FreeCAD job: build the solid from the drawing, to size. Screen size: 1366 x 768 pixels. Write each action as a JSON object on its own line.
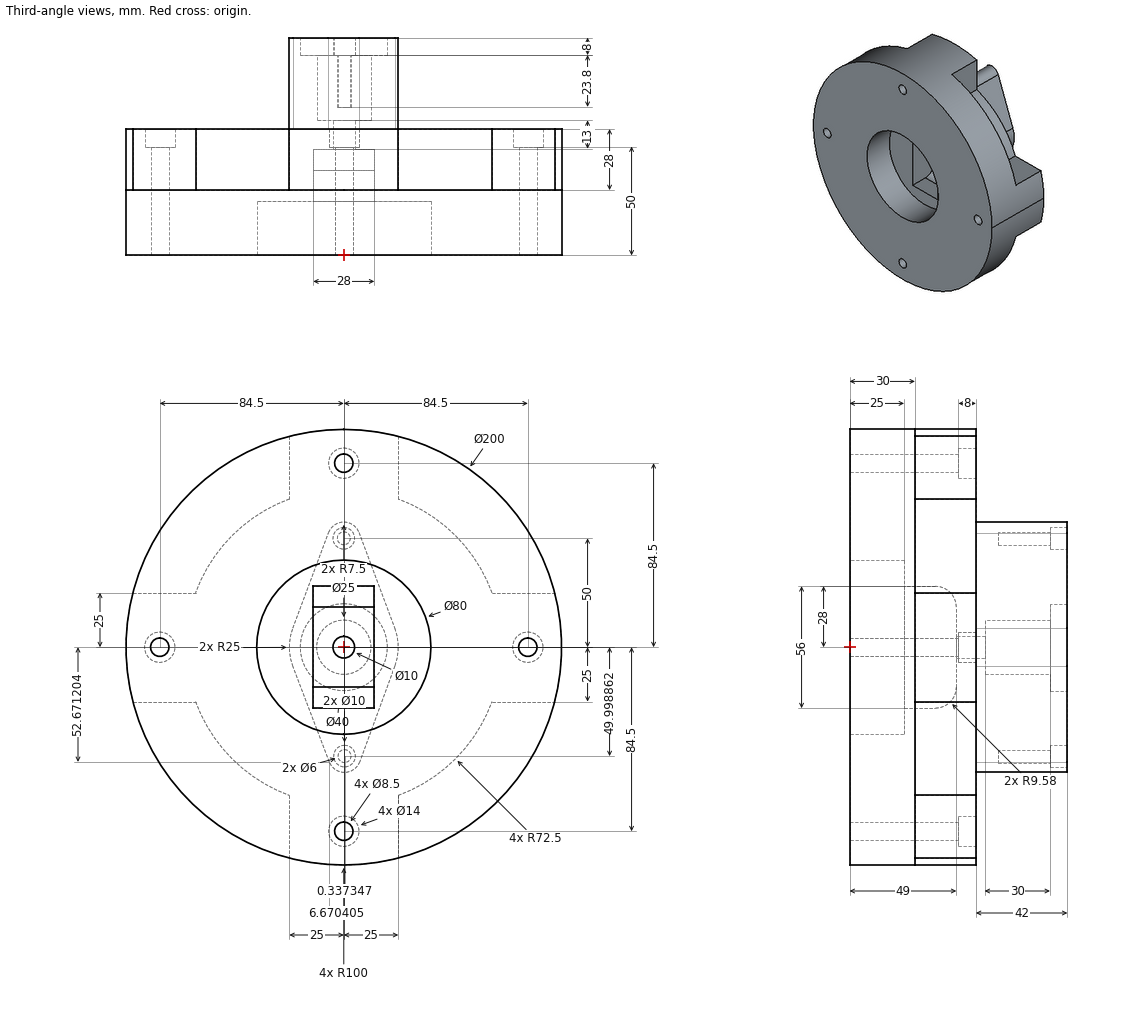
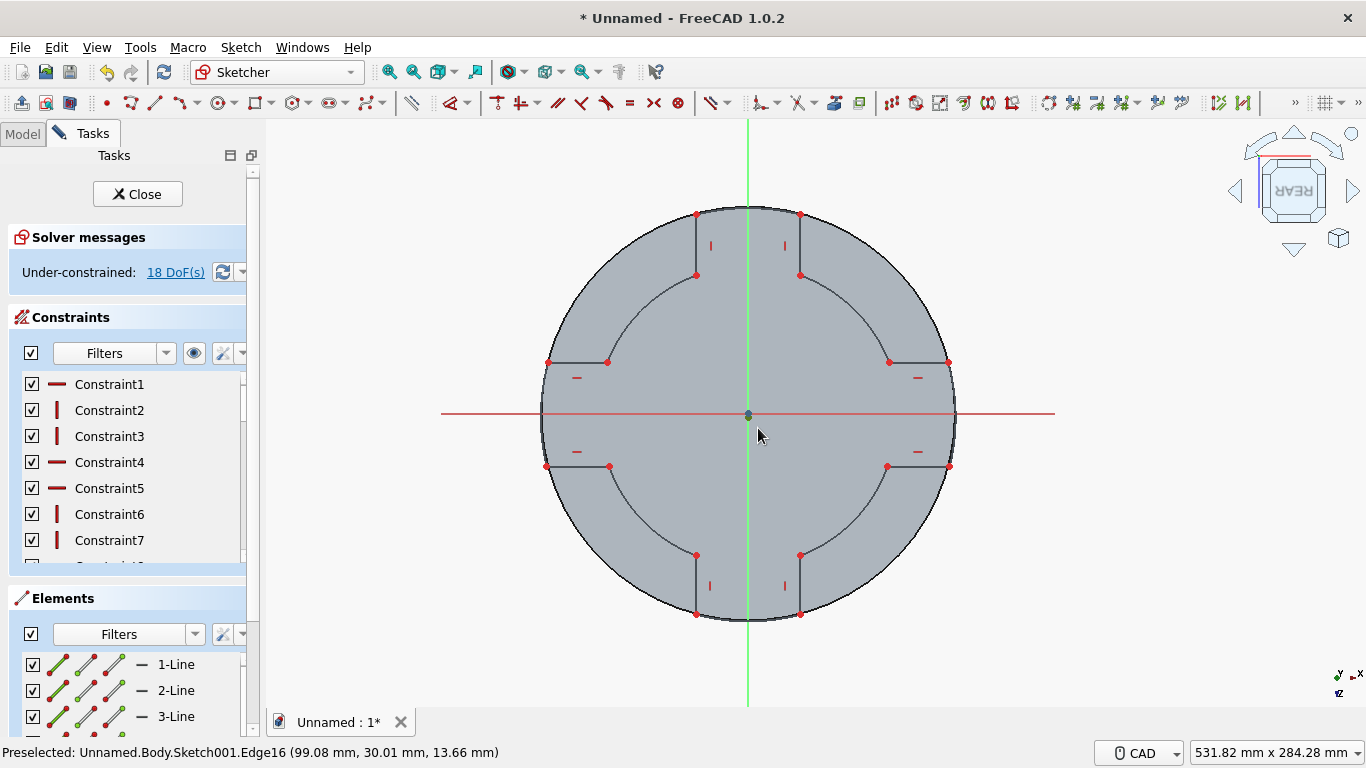
{"action": "left_click", "coordinate": [498, 104]}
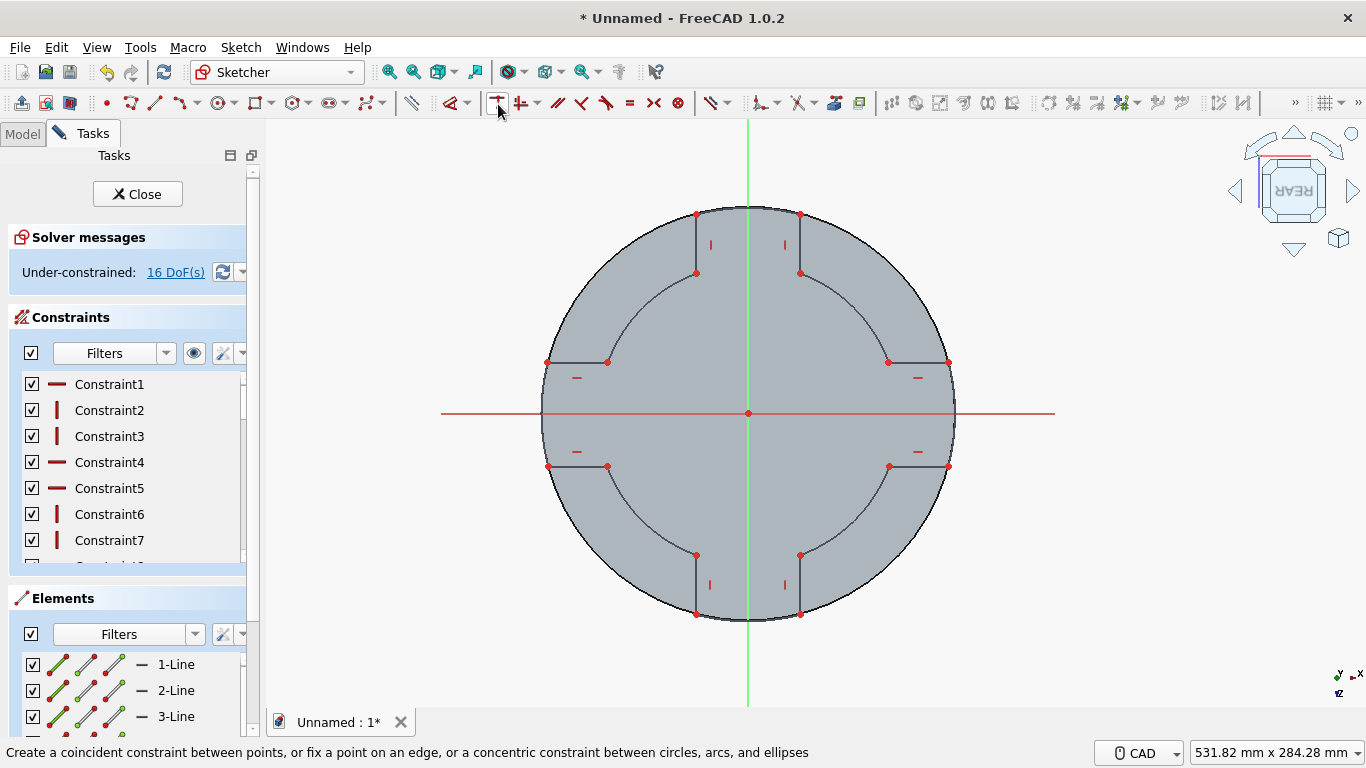
{"action": "left_click", "coordinate": [871, 328]}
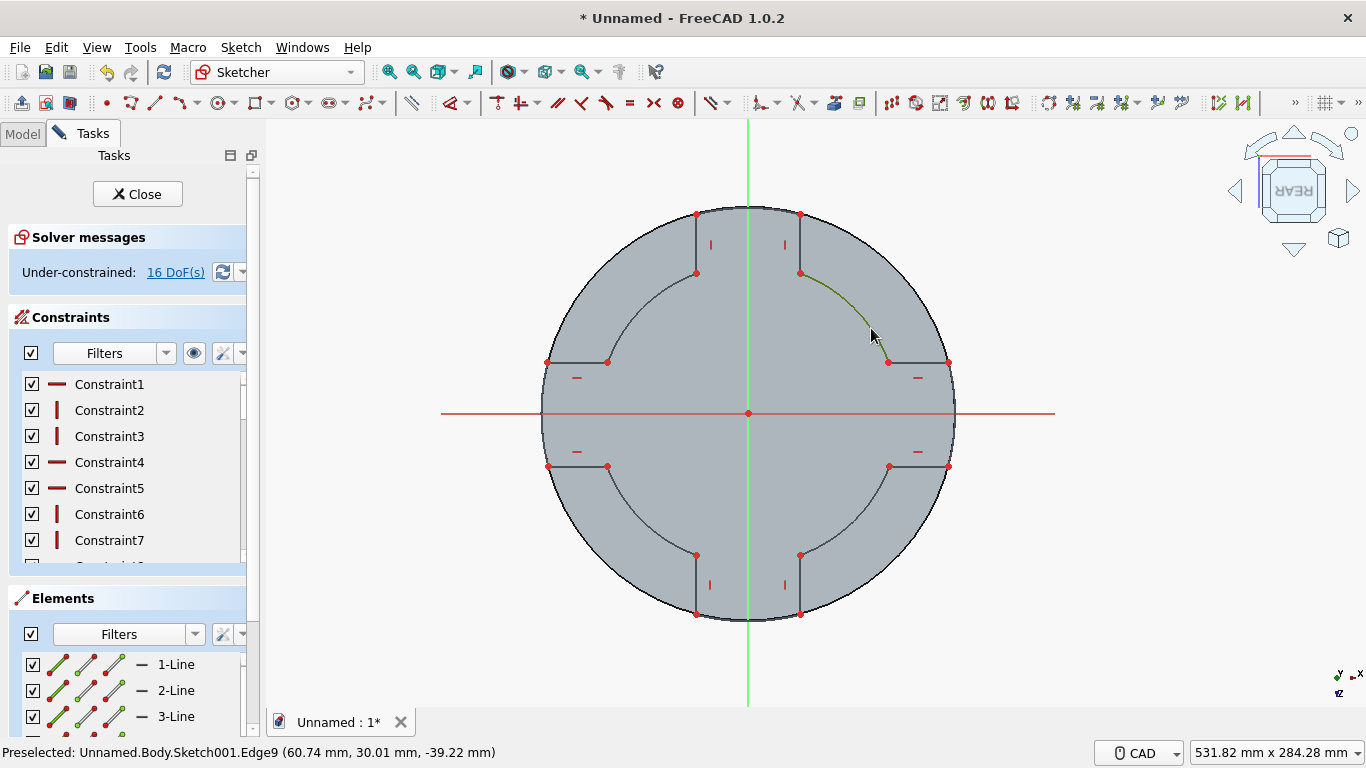
{"action": "left_click", "coordinate": [662, 292]}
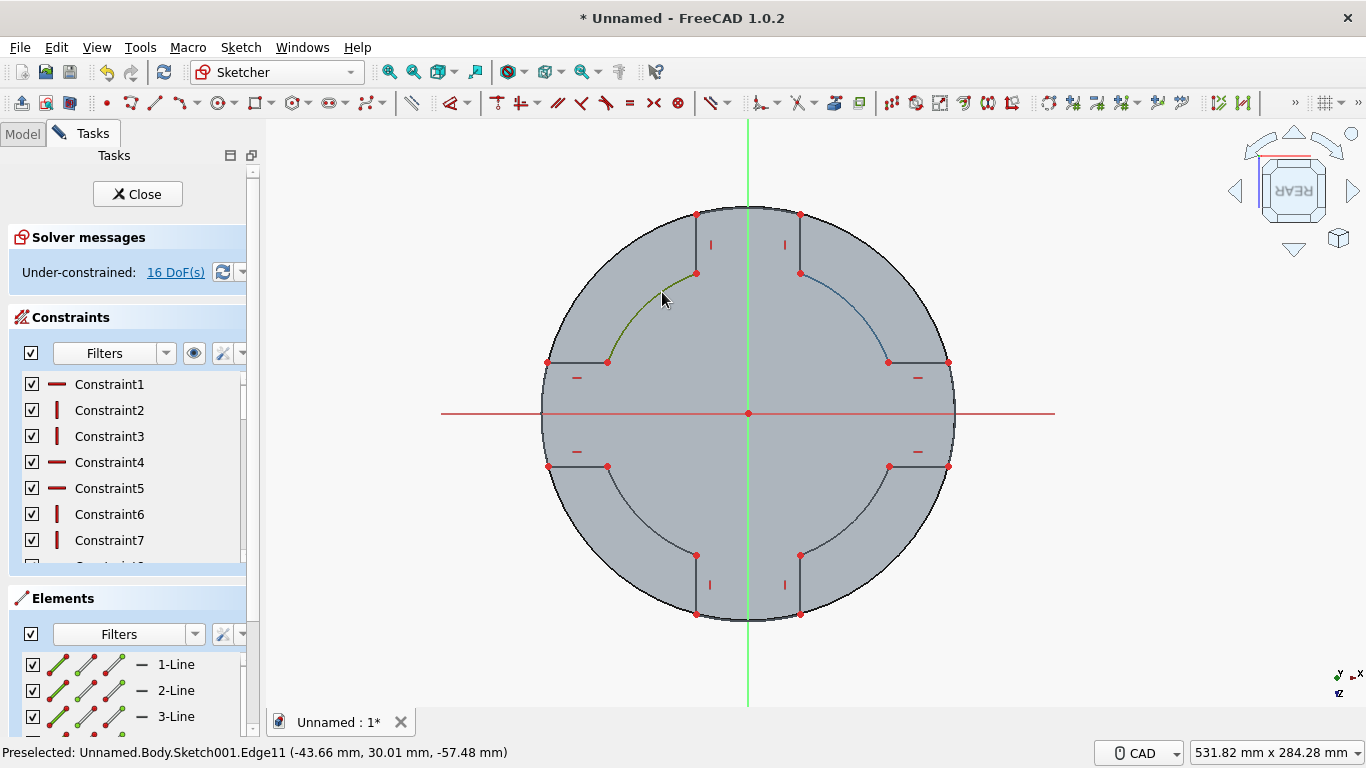
{"action": "left_click", "coordinate": [625, 501]}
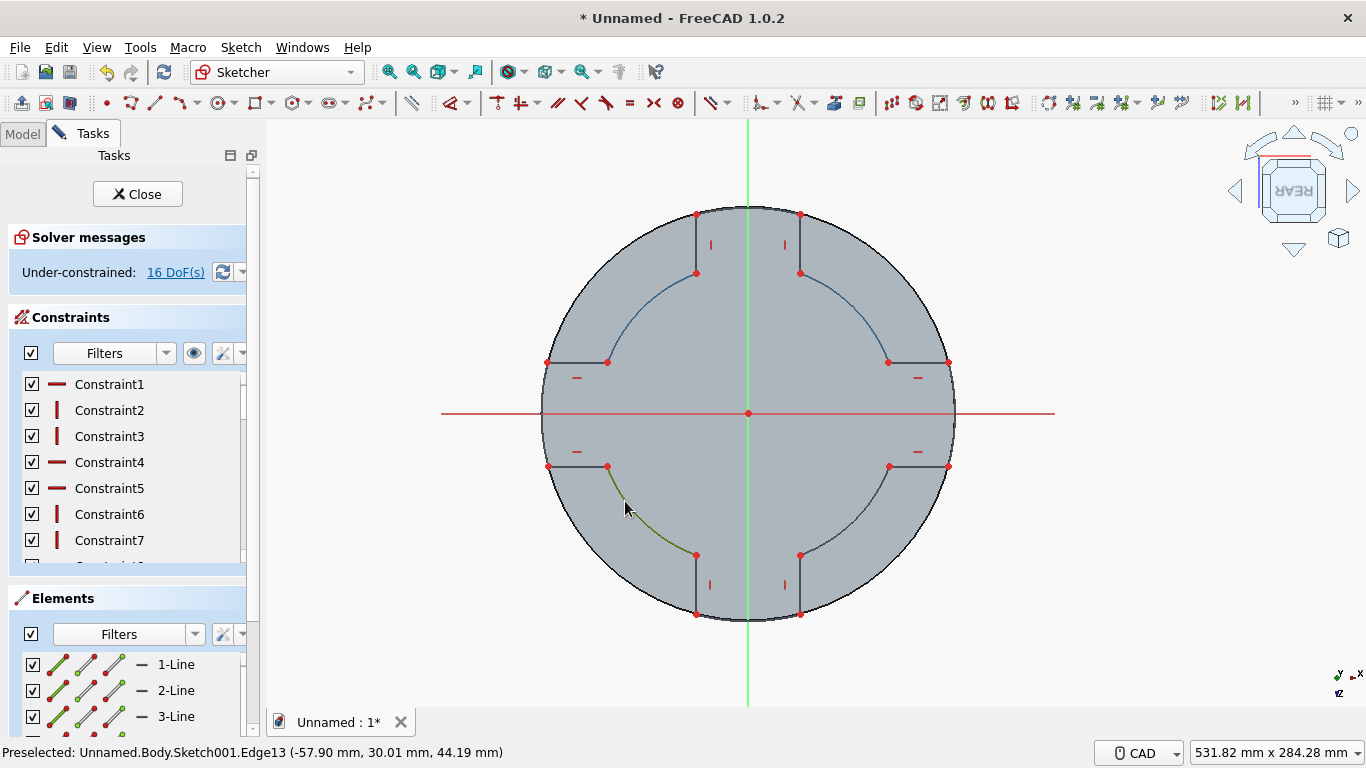
{"action": "left_click", "coordinate": [835, 537]}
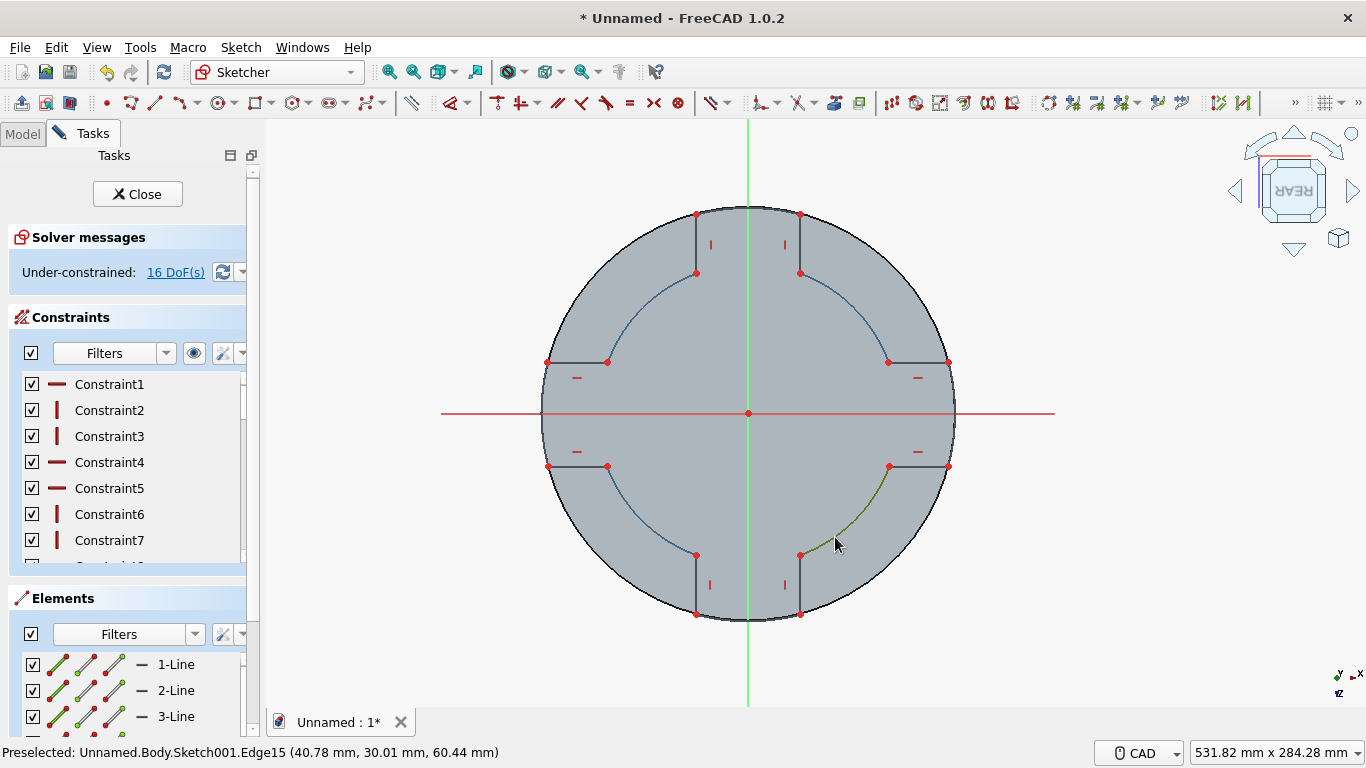
{"action": "key", "text": "e"}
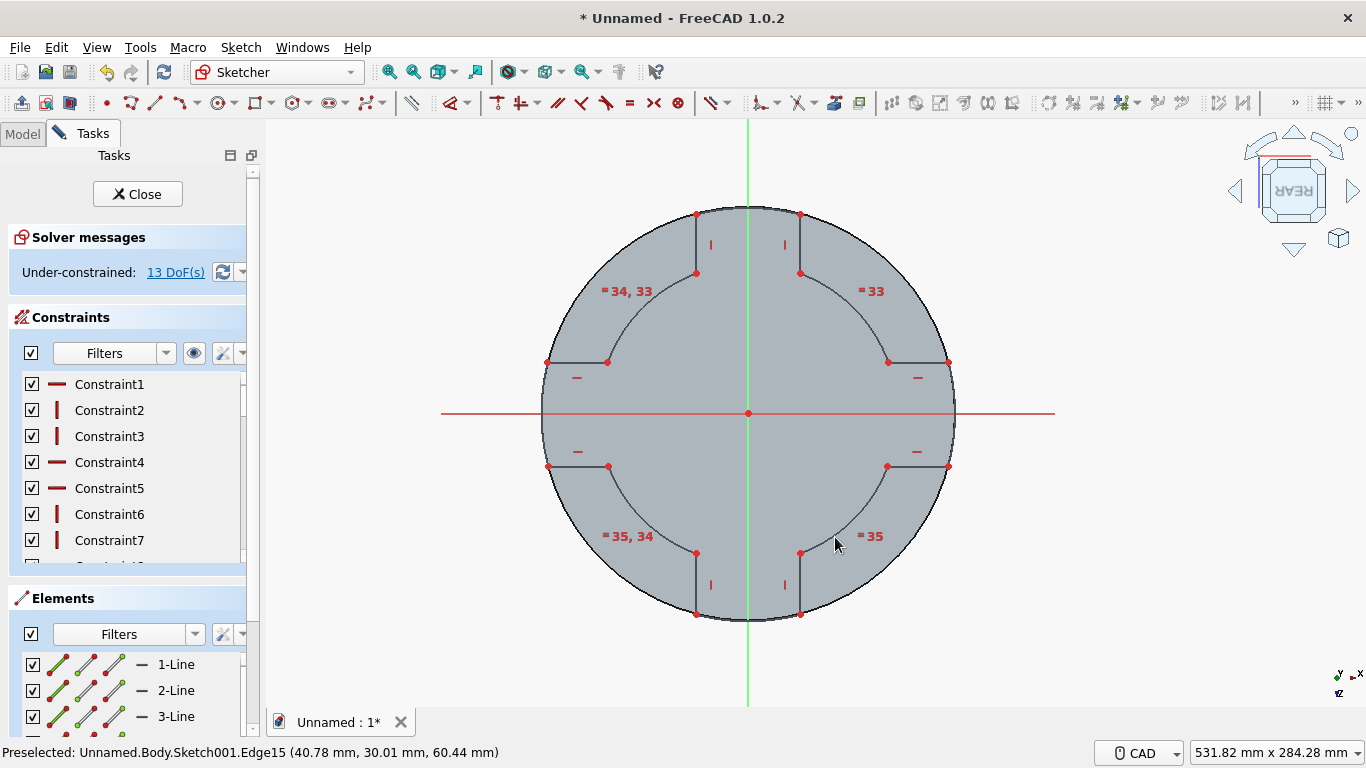
{"action": "left_click", "coordinate": [769, 209]}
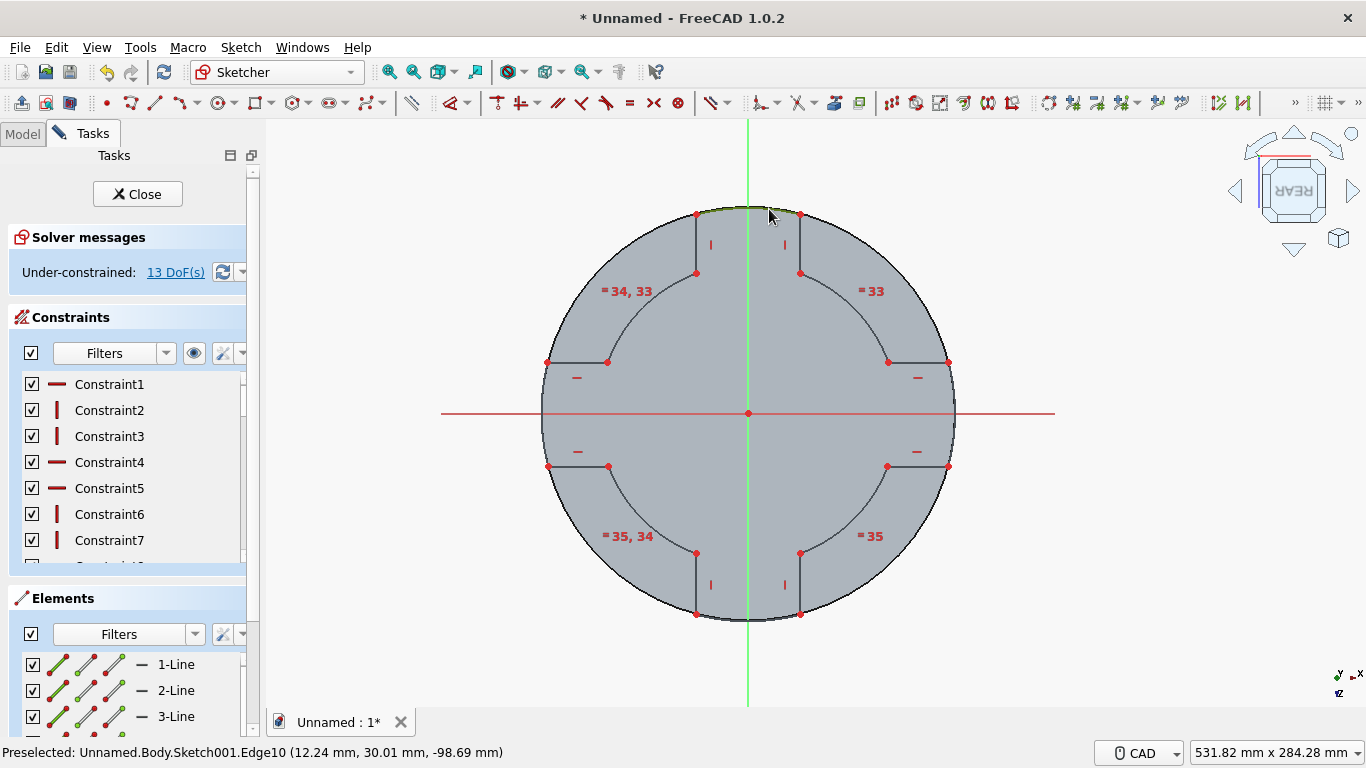
{"action": "left_click", "coordinate": [542, 394]}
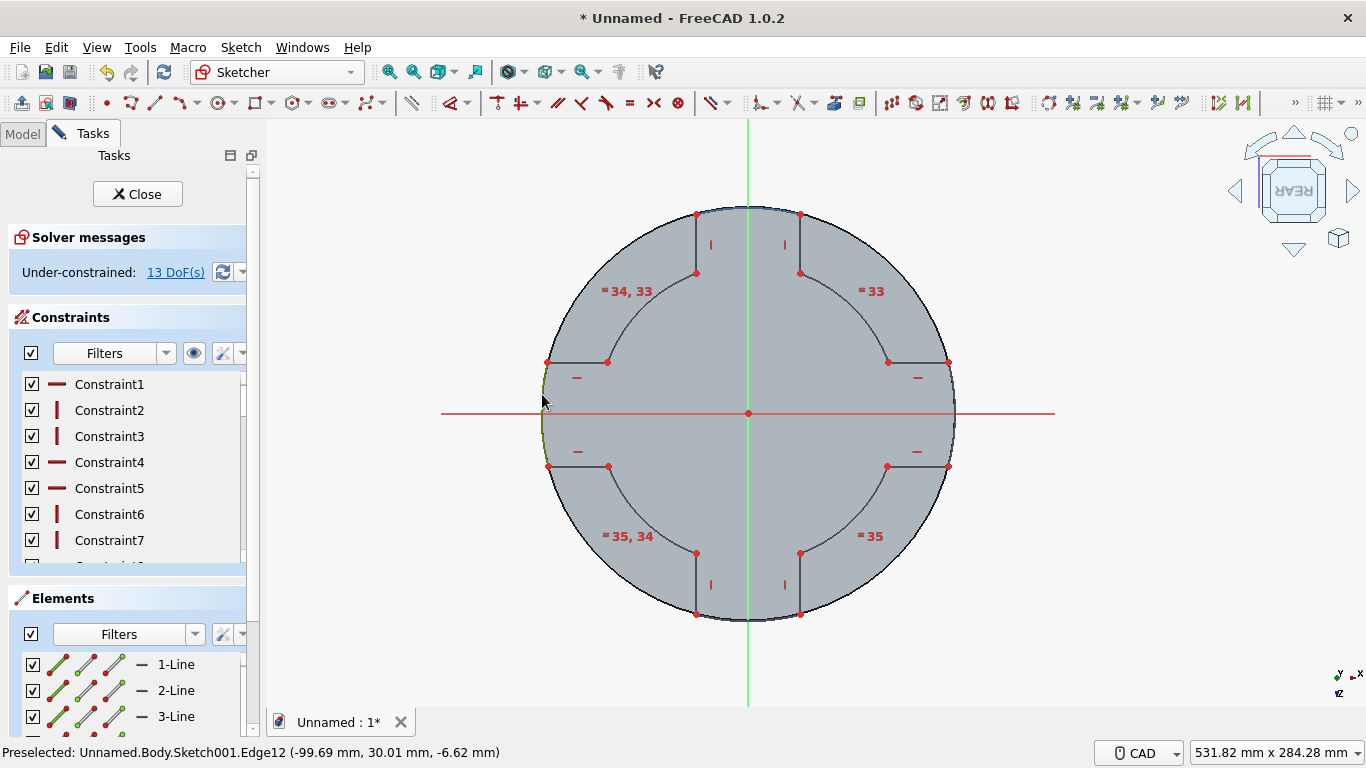
{"action": "left_click", "coordinate": [727, 620]}